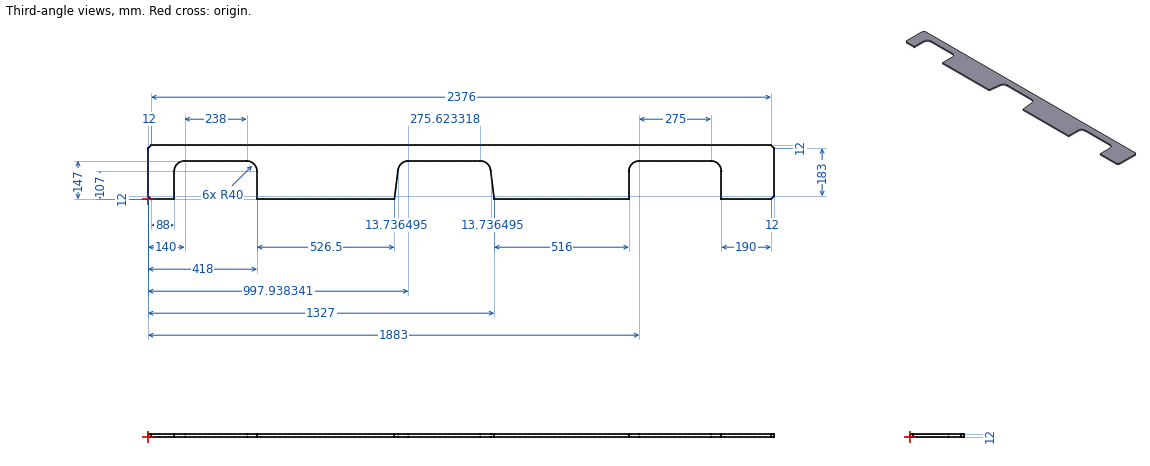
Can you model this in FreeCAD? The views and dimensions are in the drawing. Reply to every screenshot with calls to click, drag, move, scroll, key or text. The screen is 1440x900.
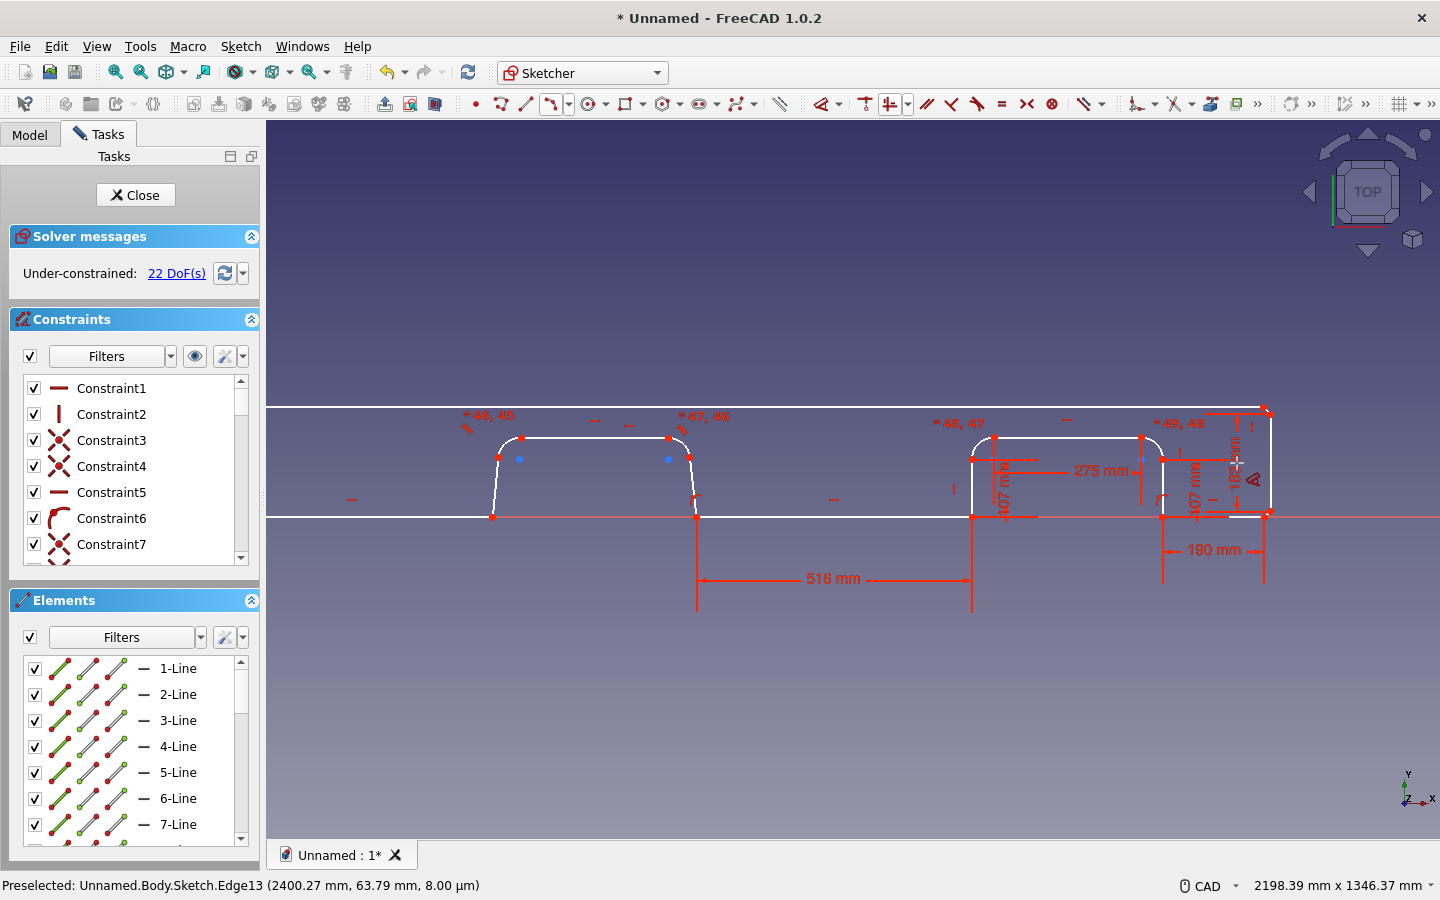
scroll(973, 501, down, 3)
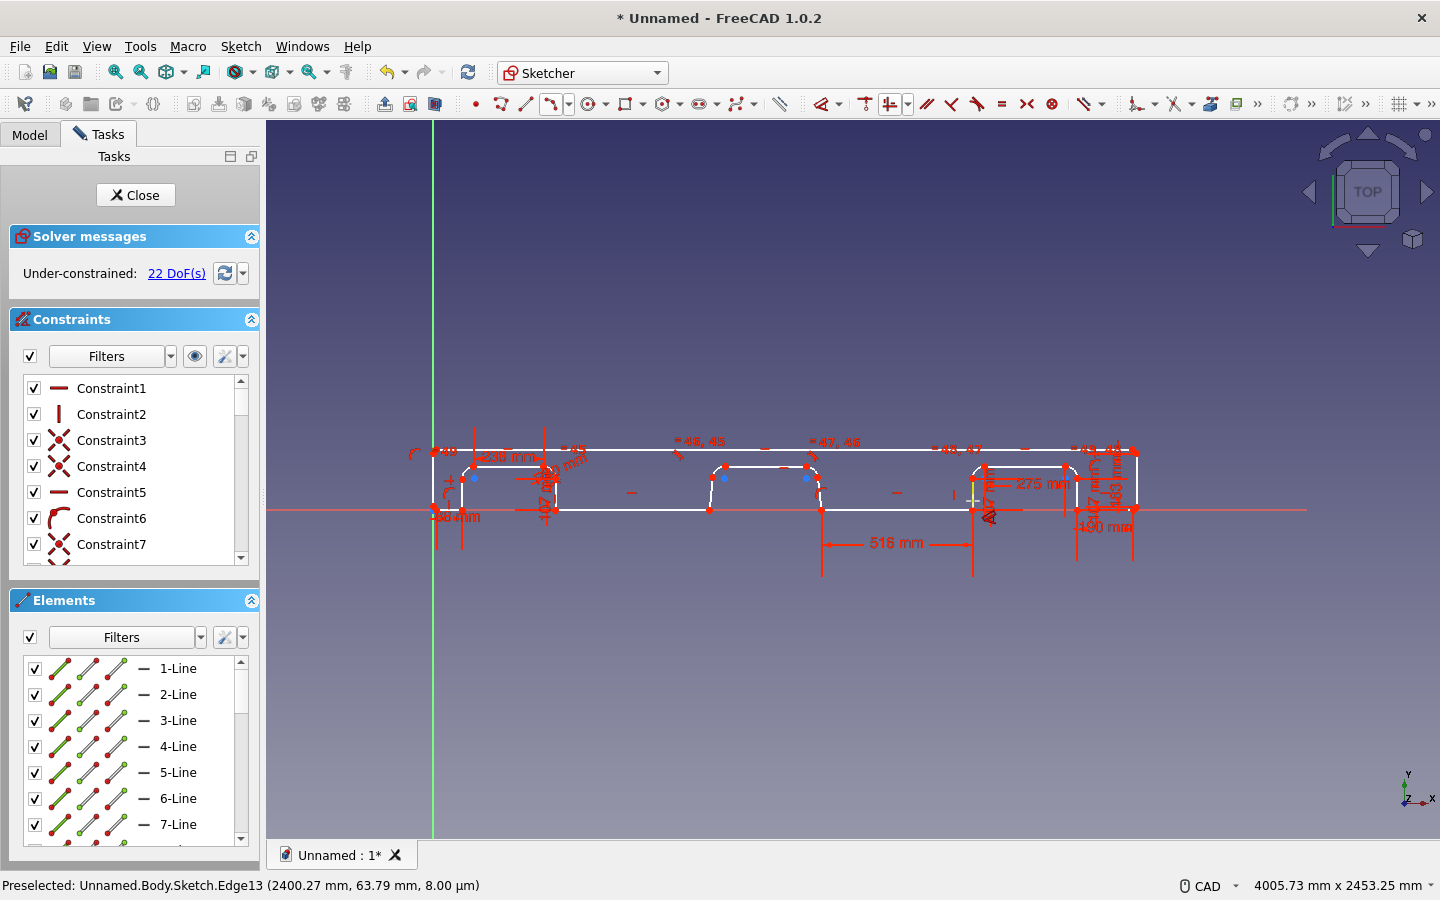
click(433, 469)
click(399, 480)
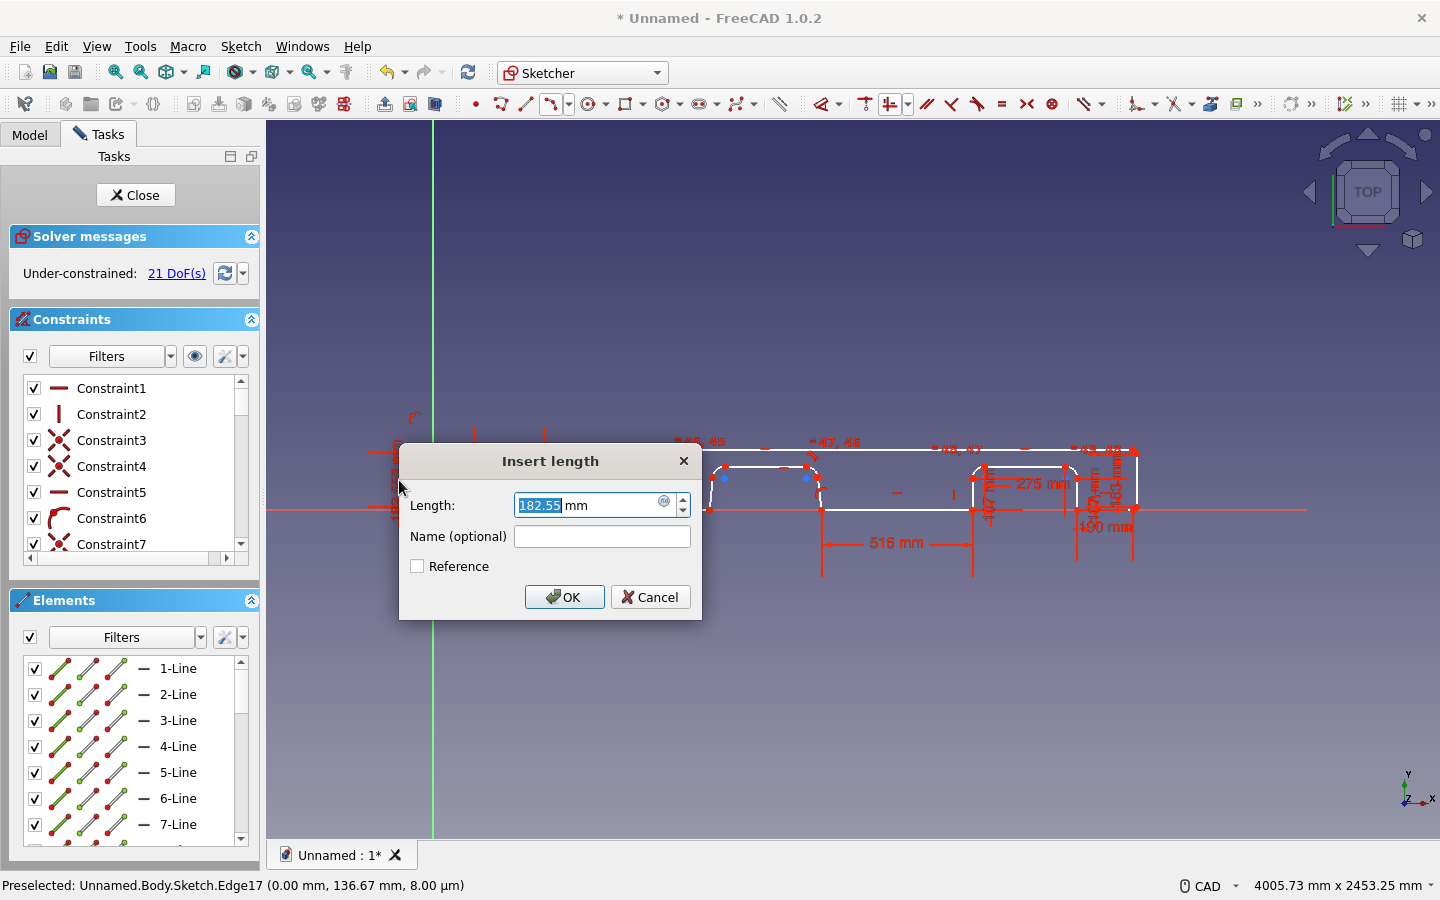
text(183)
key(Return)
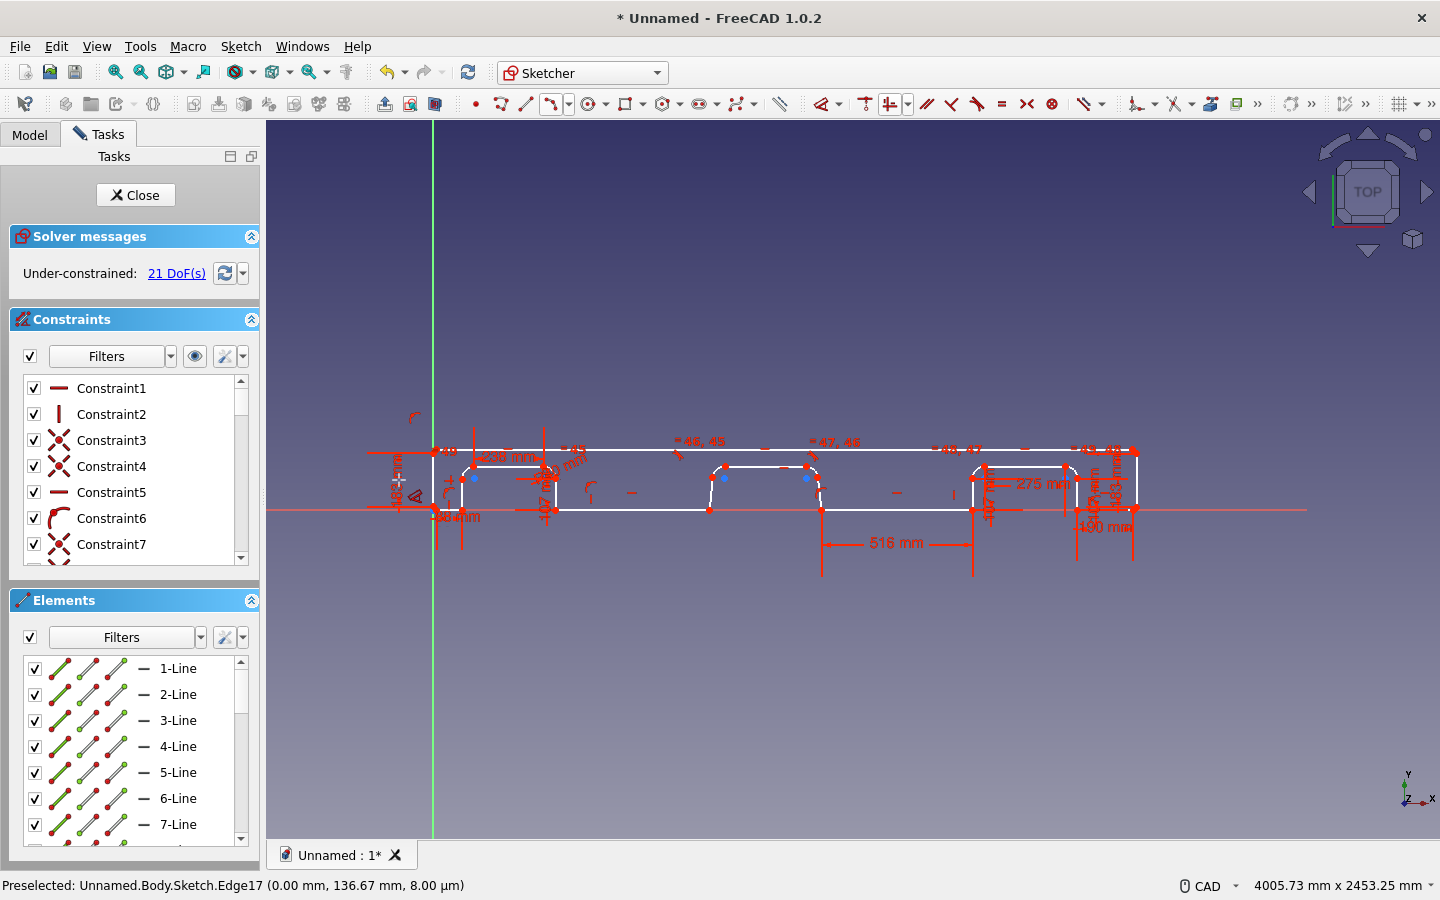
scroll(462, 501, up, 3)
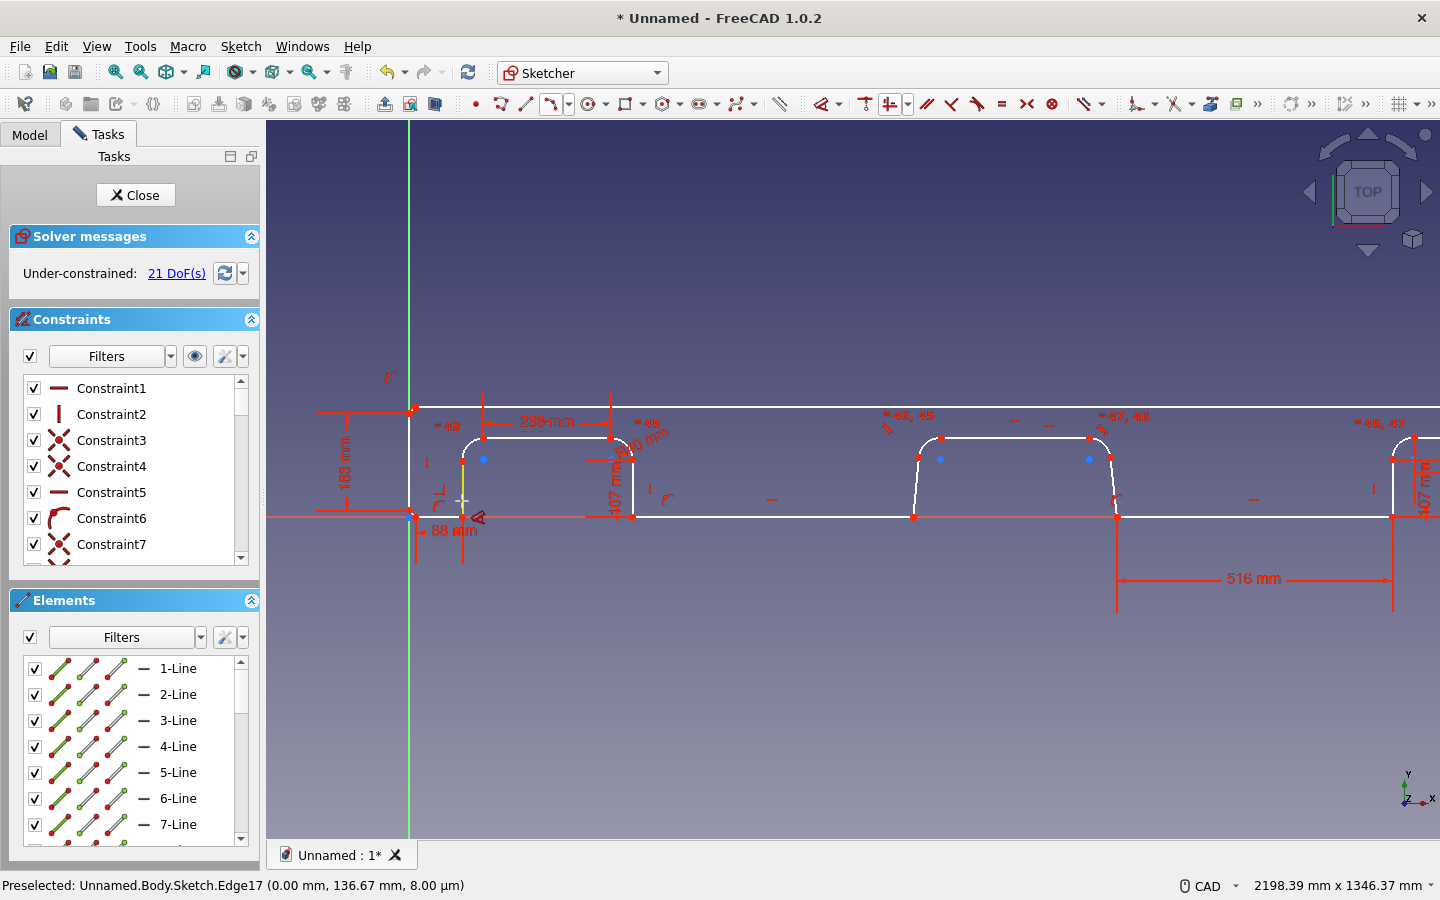
click(463, 501)
click(429, 489)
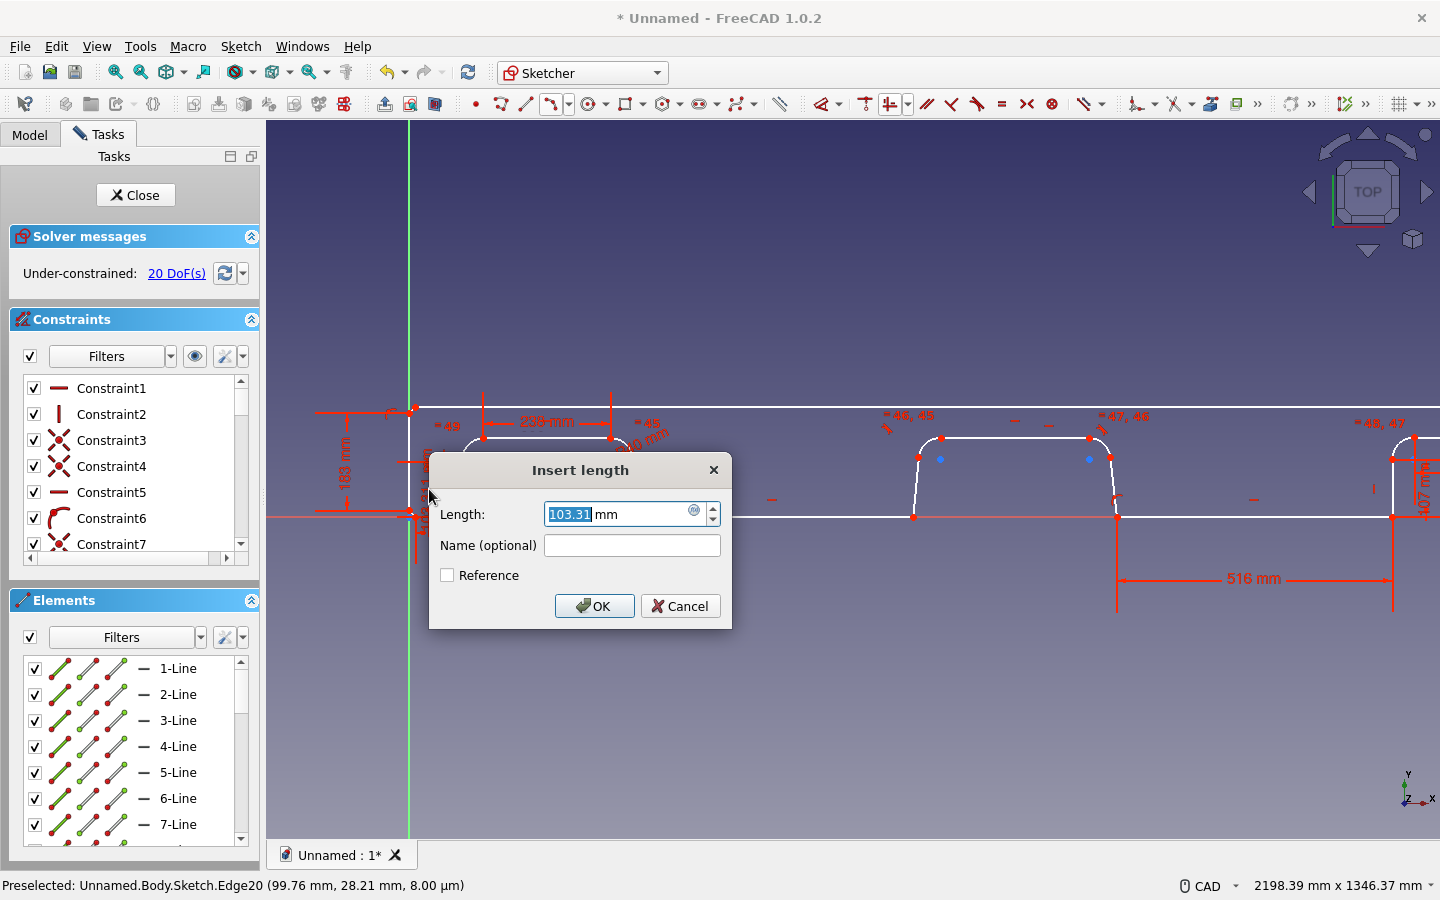
text(107)
key(Return)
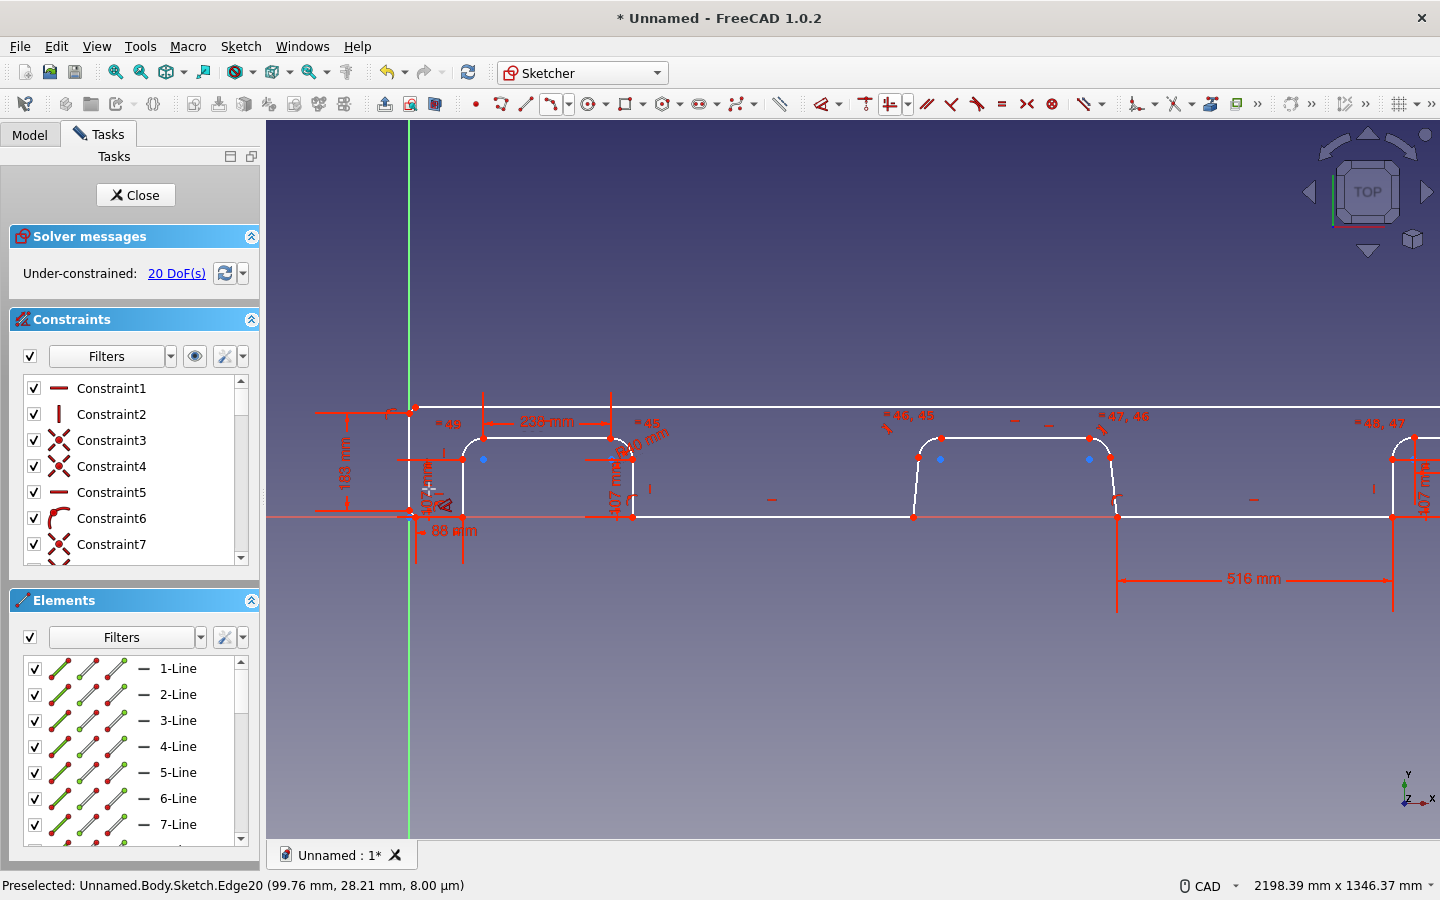
scroll(461, 501, down, 3)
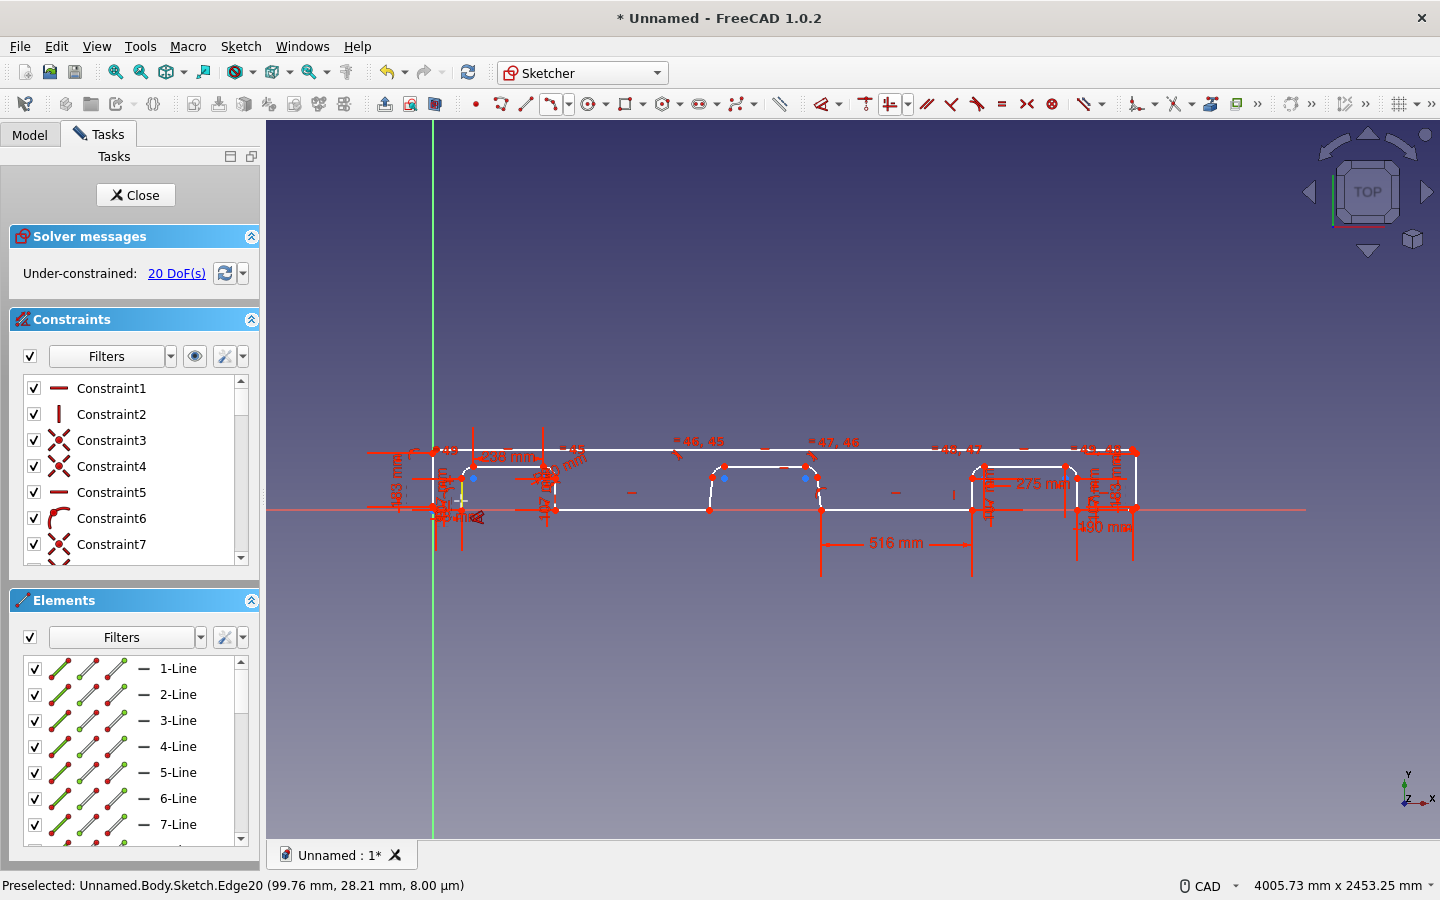
scroll(1136, 507, up, 13)